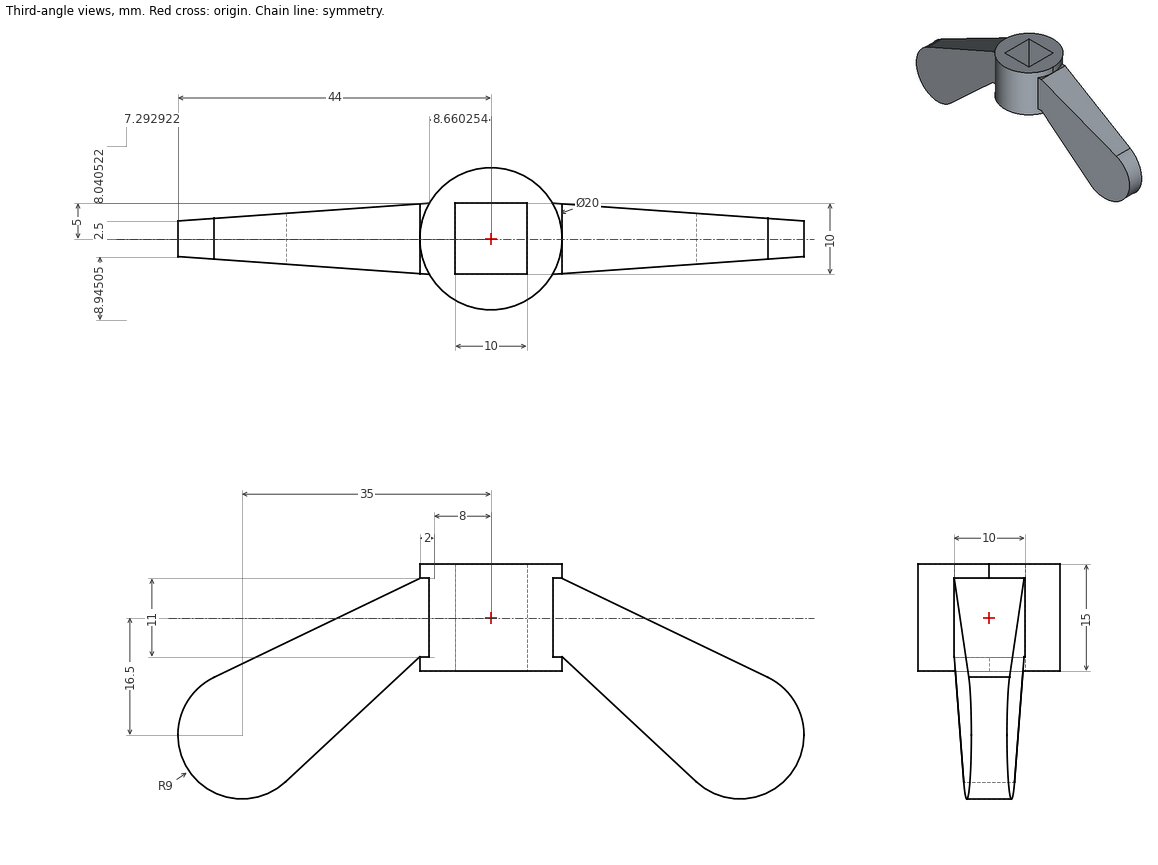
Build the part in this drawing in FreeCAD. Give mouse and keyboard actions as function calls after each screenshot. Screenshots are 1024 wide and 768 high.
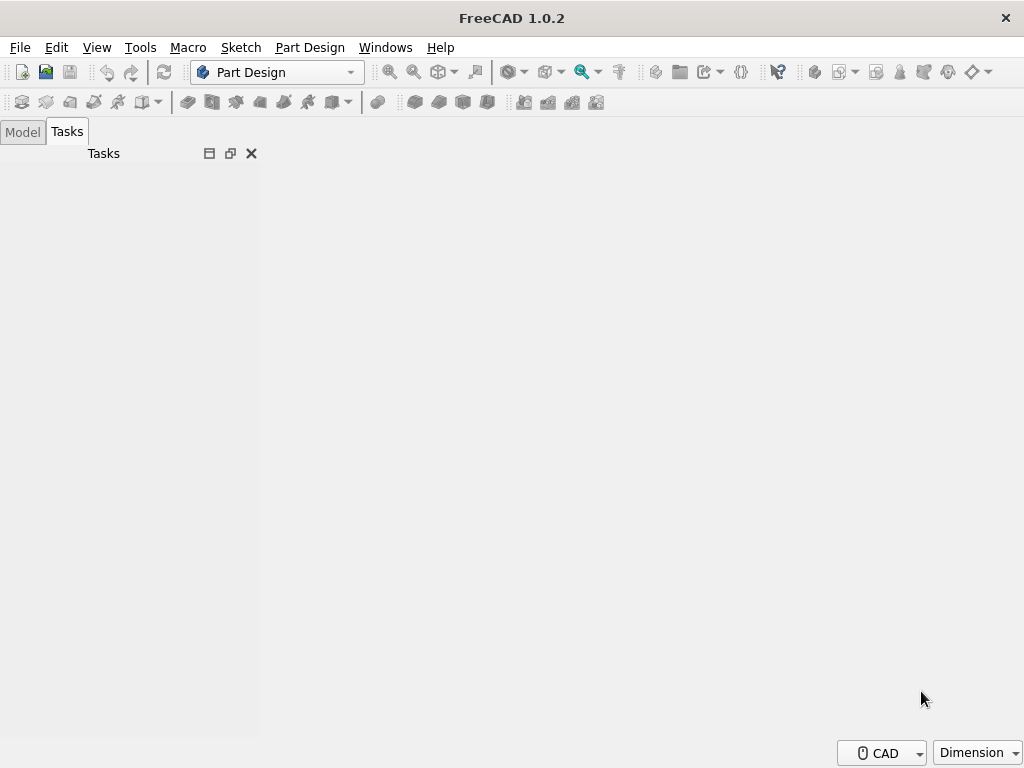
click(22, 72)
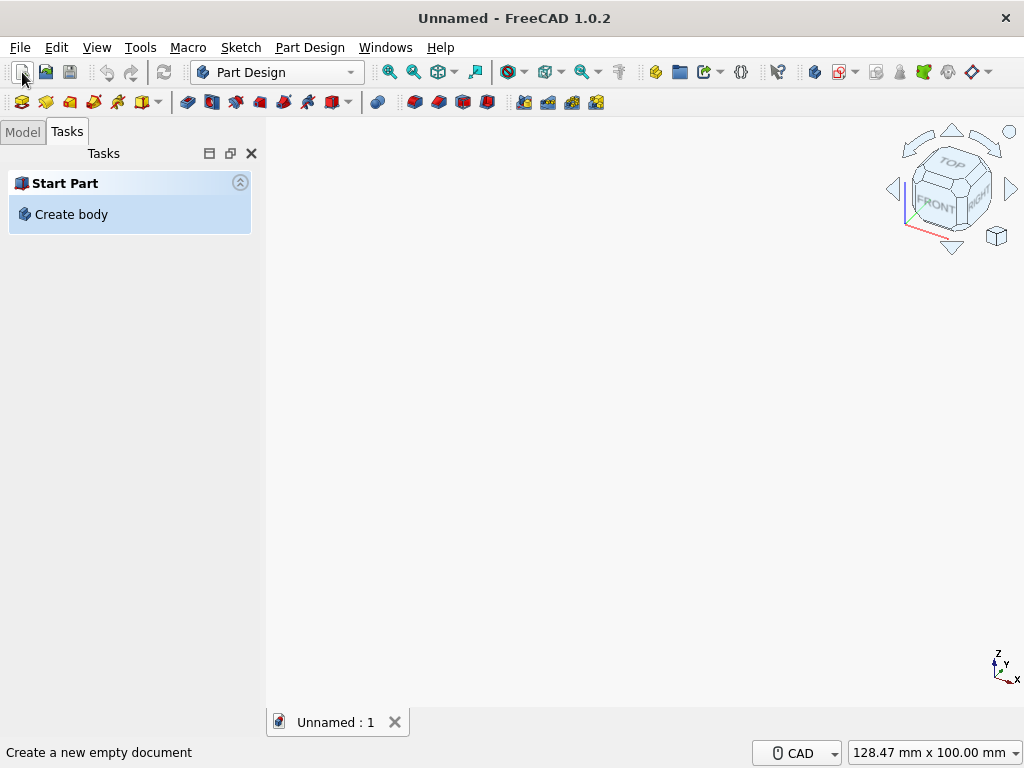
click(840, 72)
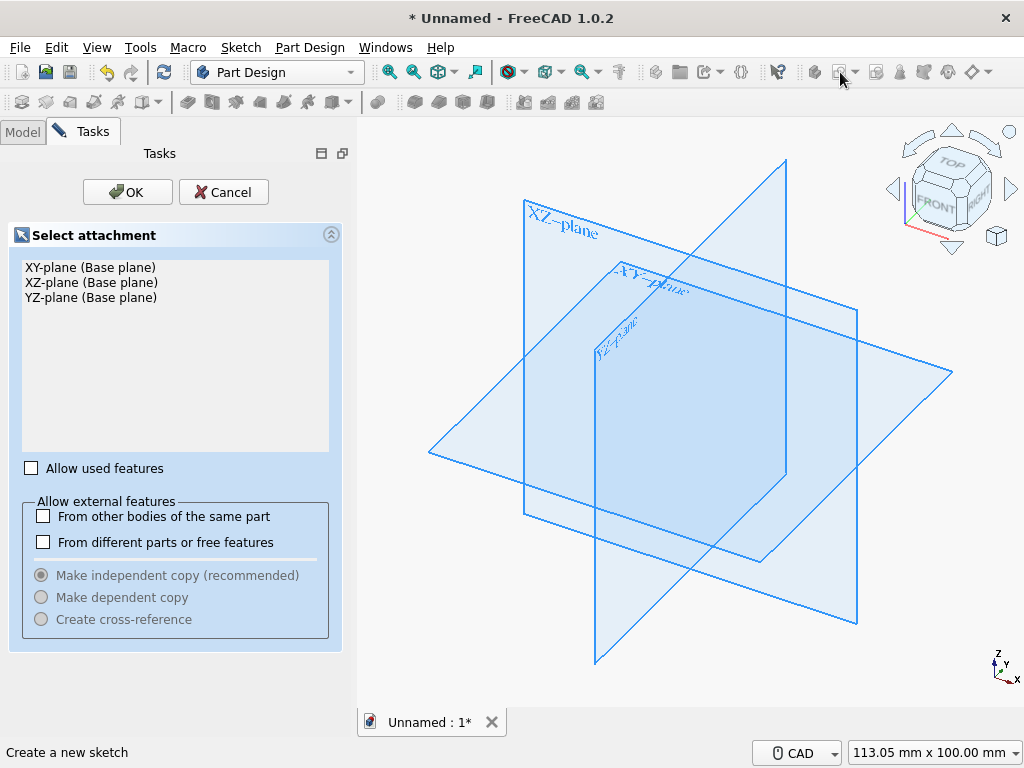
click(82, 268)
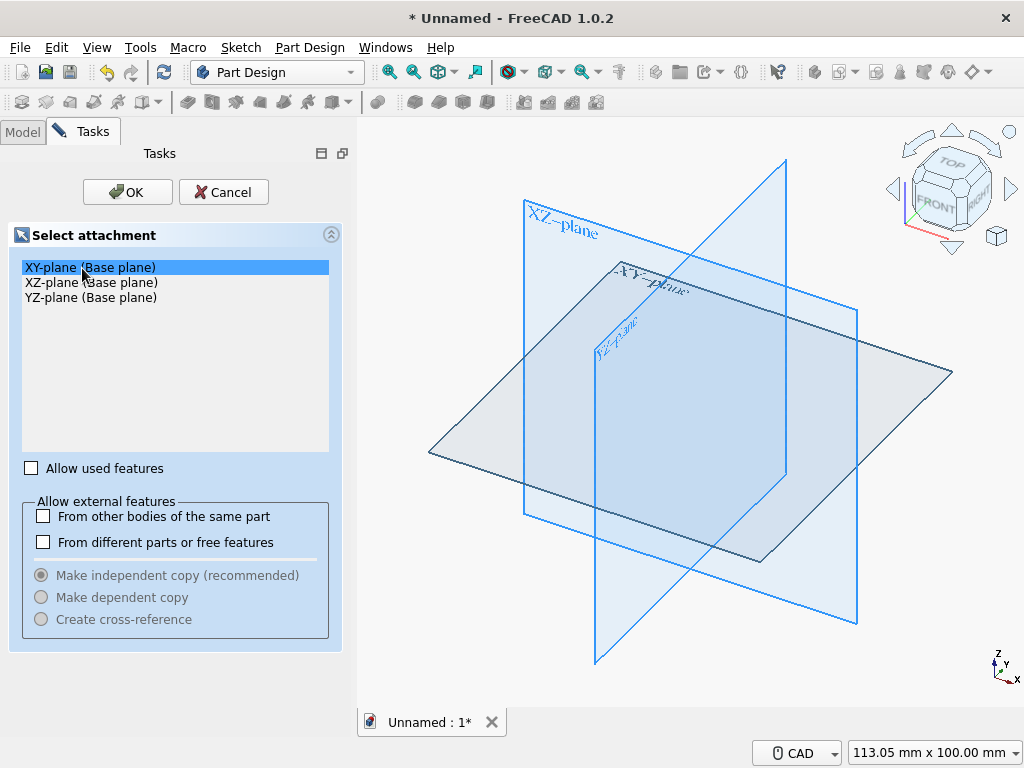
click(128, 192)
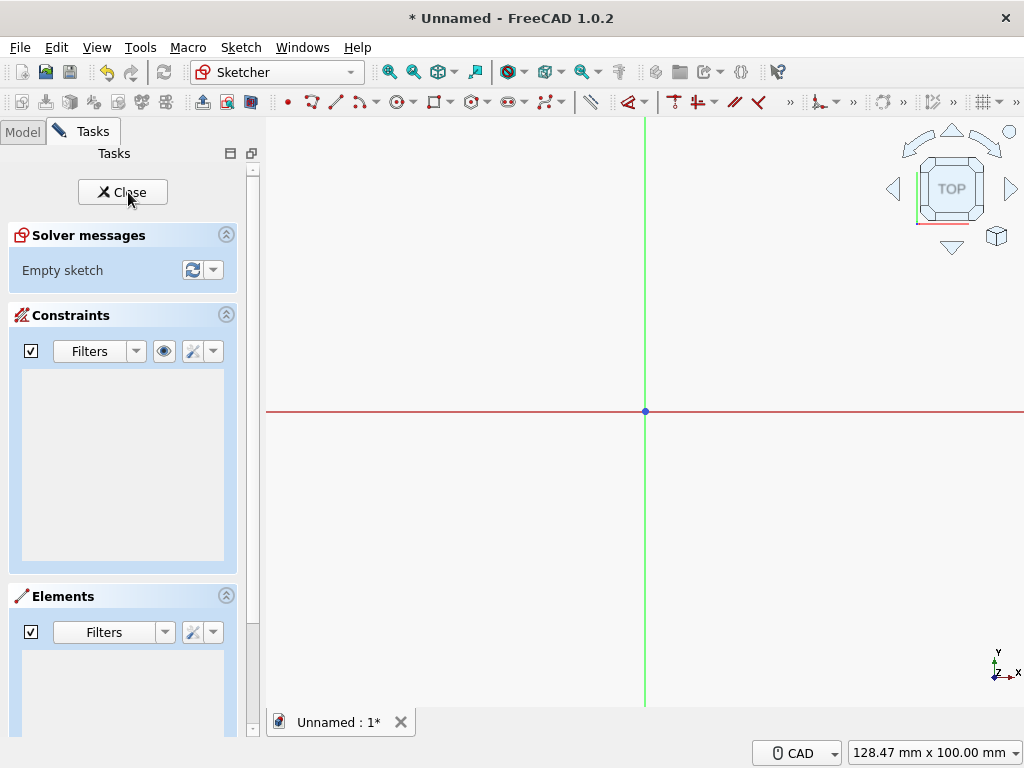
scroll(675, 412, up, 6)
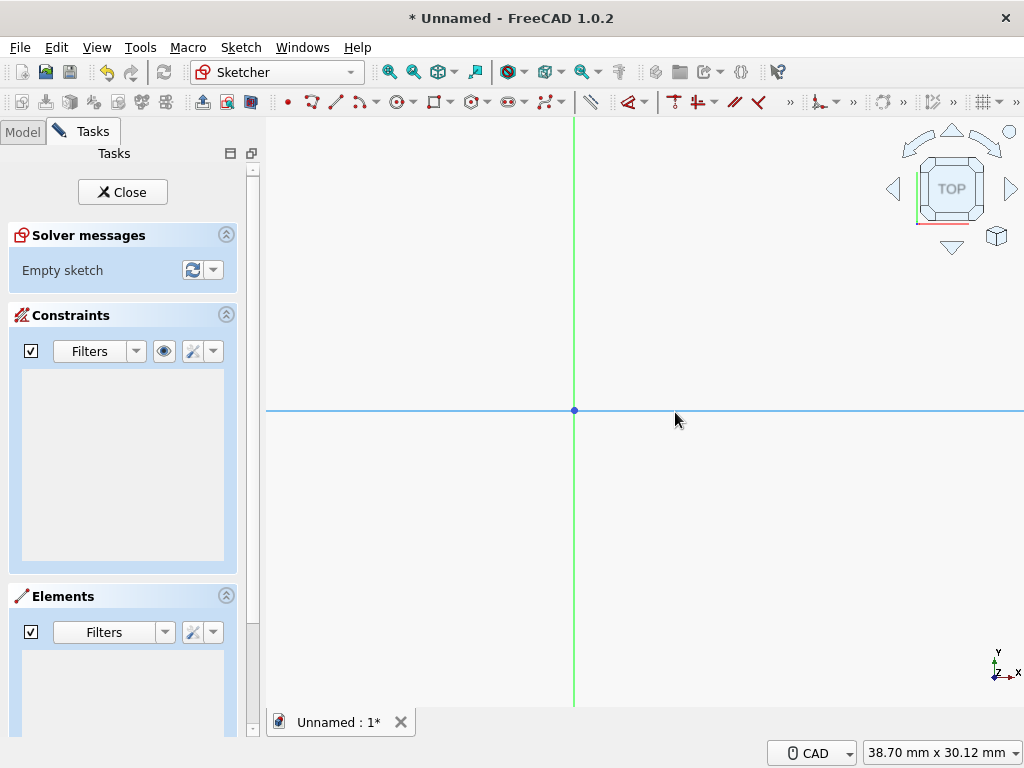
key(g)
key(v)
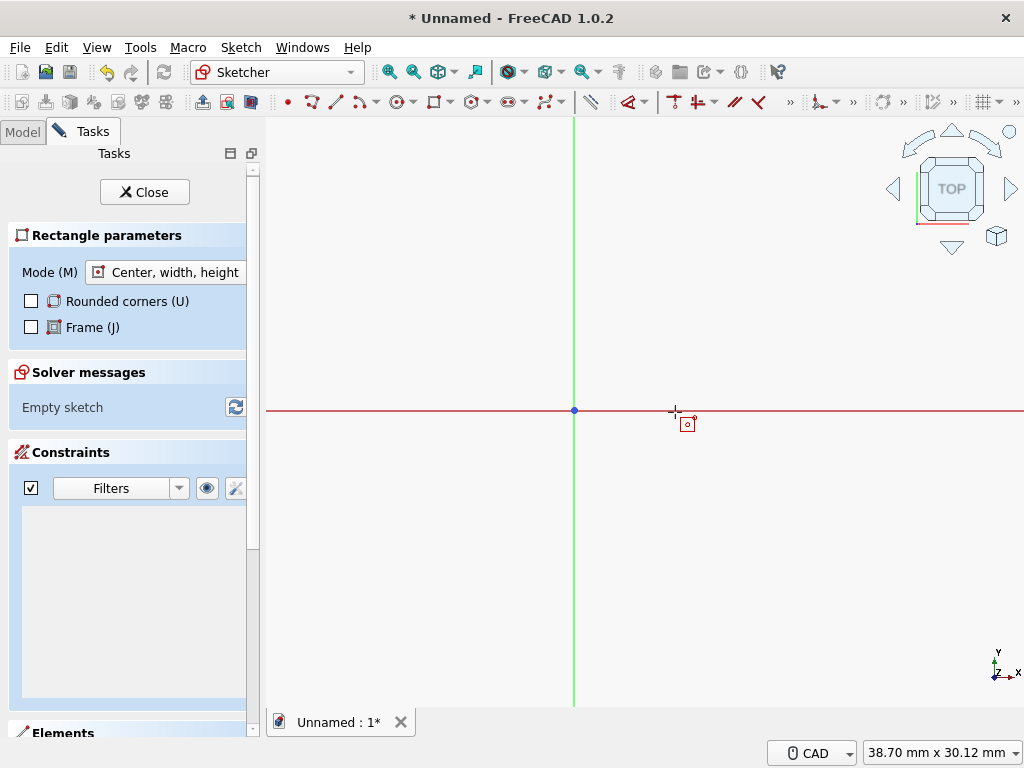
click(574, 411)
move(672, 313)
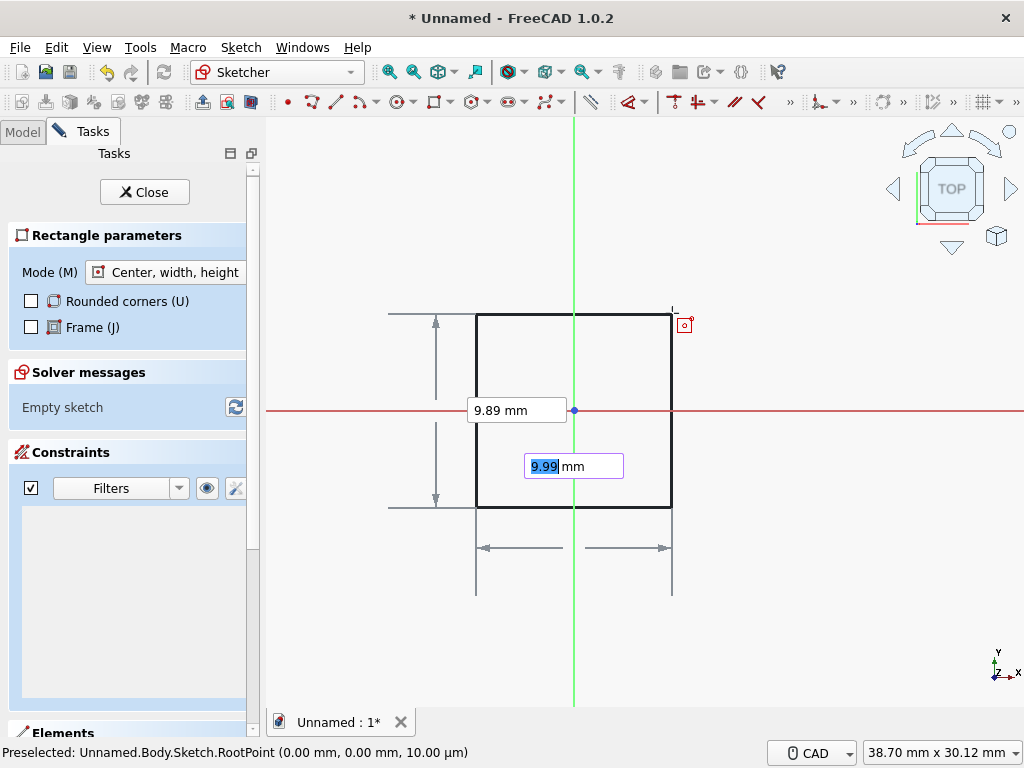
text(10)
key(Tab)
text(10)
key(Return)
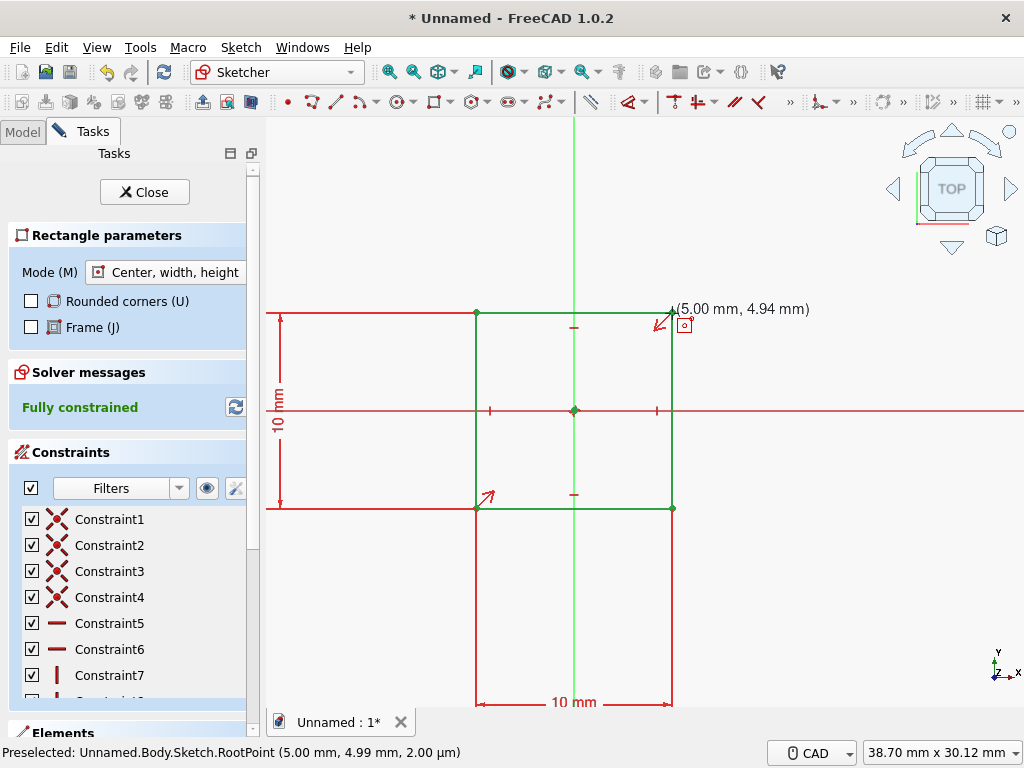
click(398, 102)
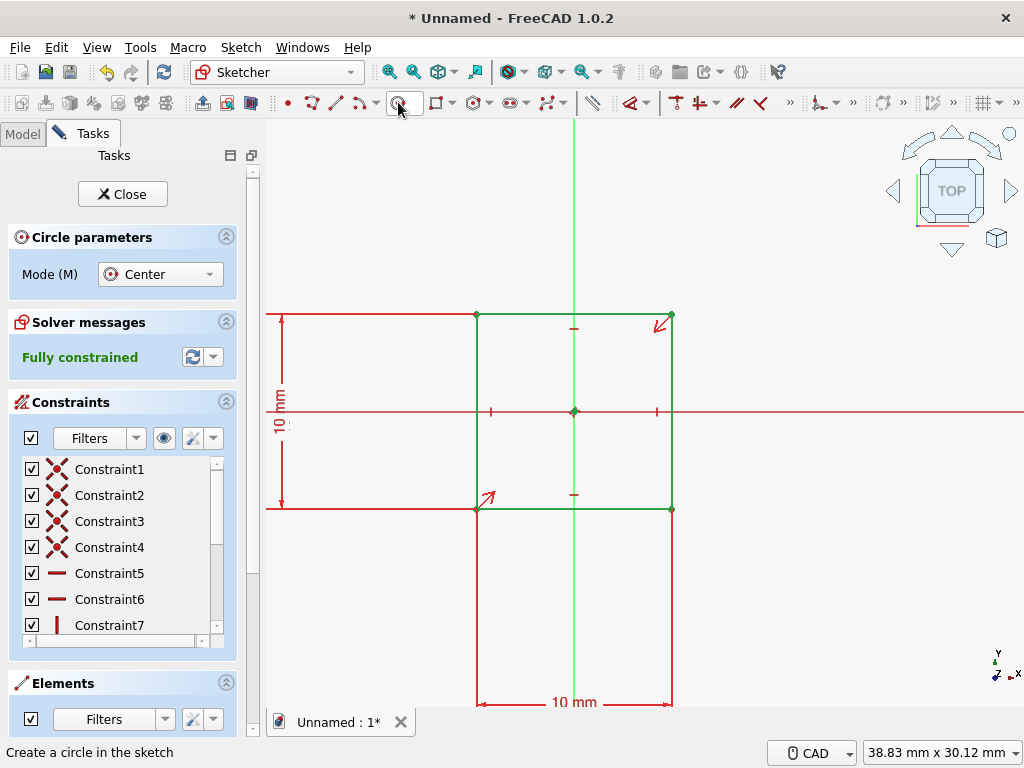
click(574, 412)
move(712, 274)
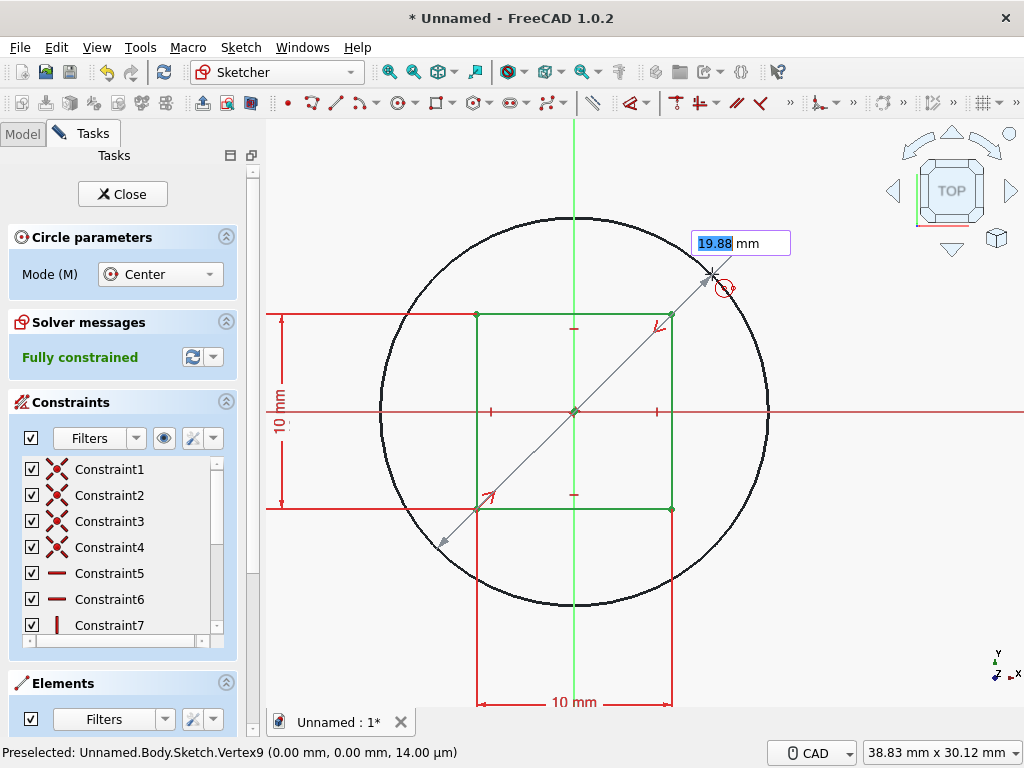
text(20)
key(Return)
key(Escape)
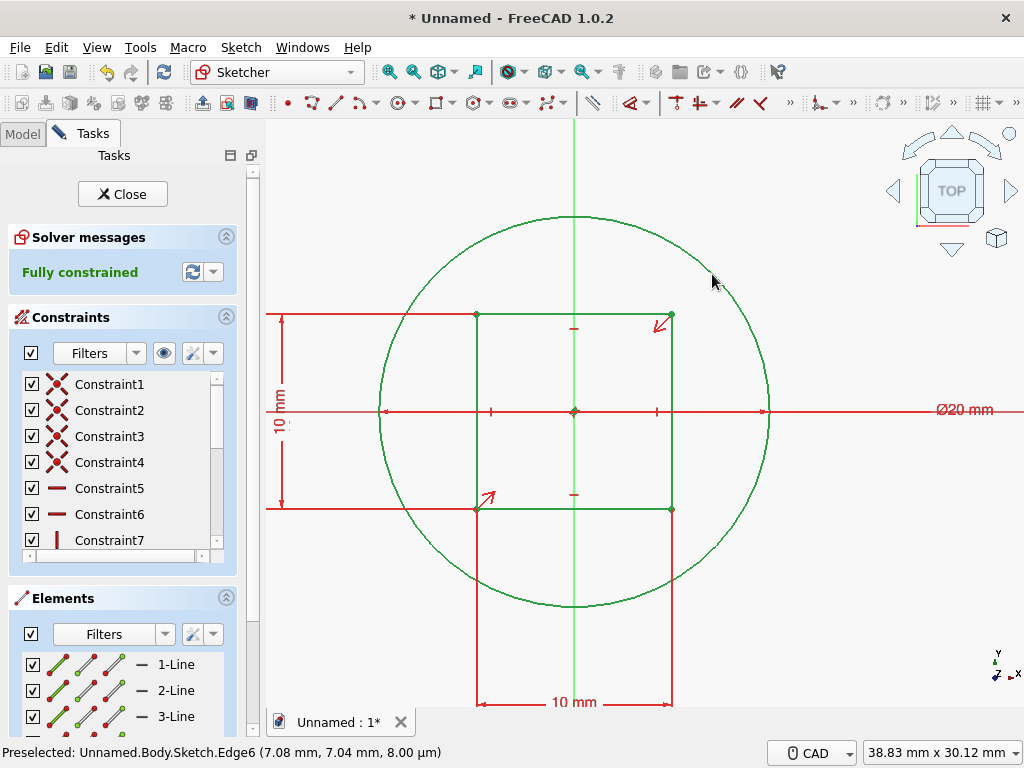
click(123, 194)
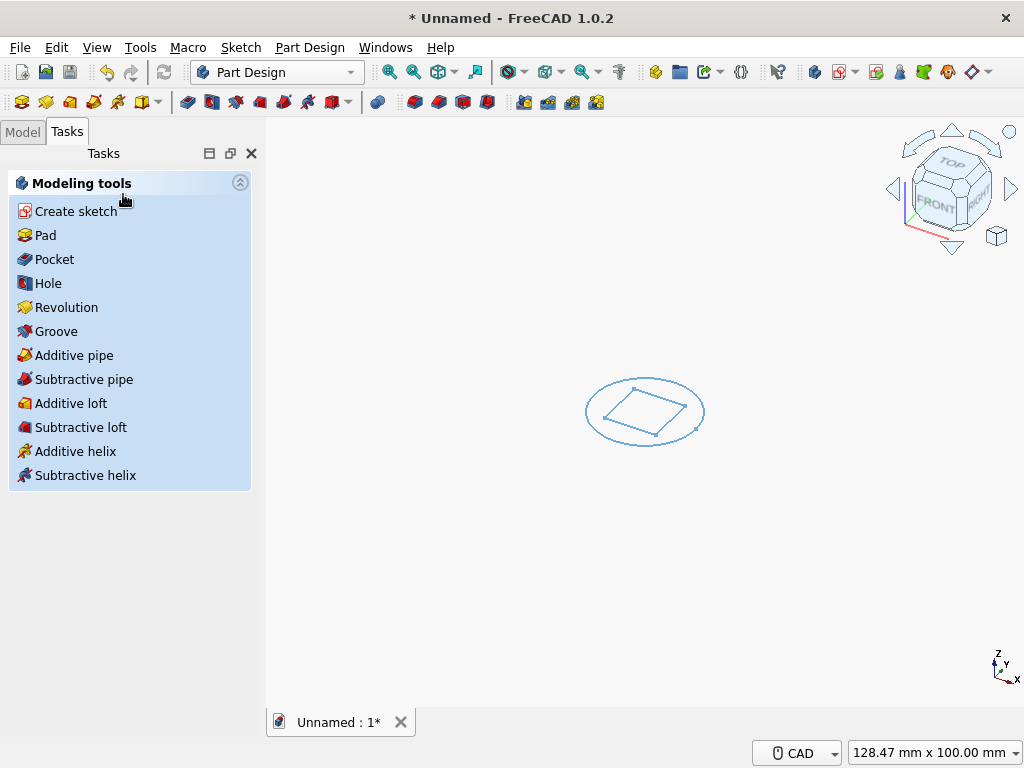
click(22, 102)